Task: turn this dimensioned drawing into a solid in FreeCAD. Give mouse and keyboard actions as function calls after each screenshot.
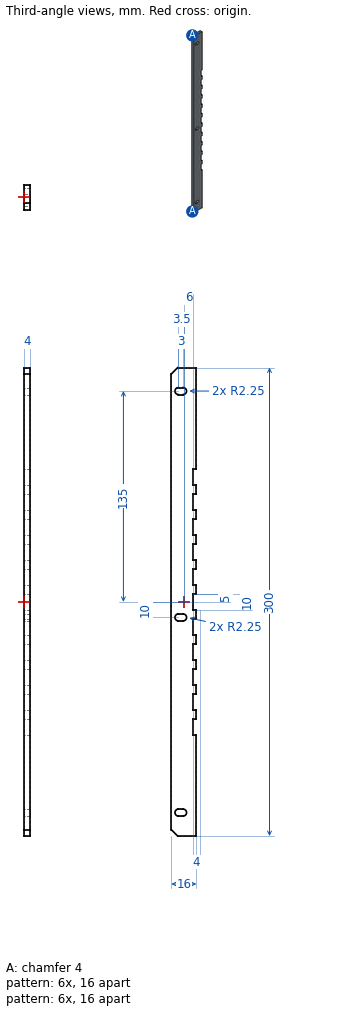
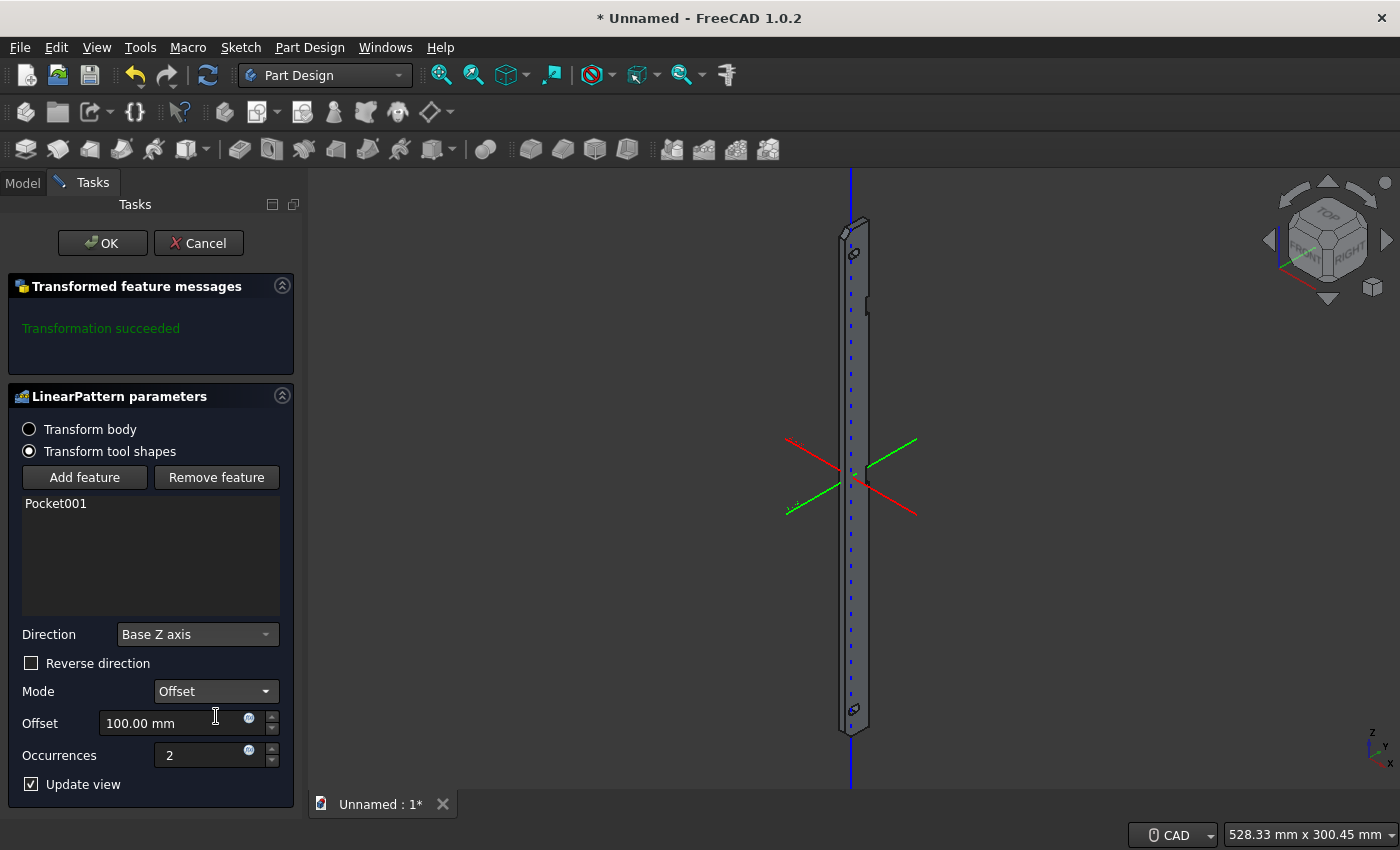
triple_click(182, 723)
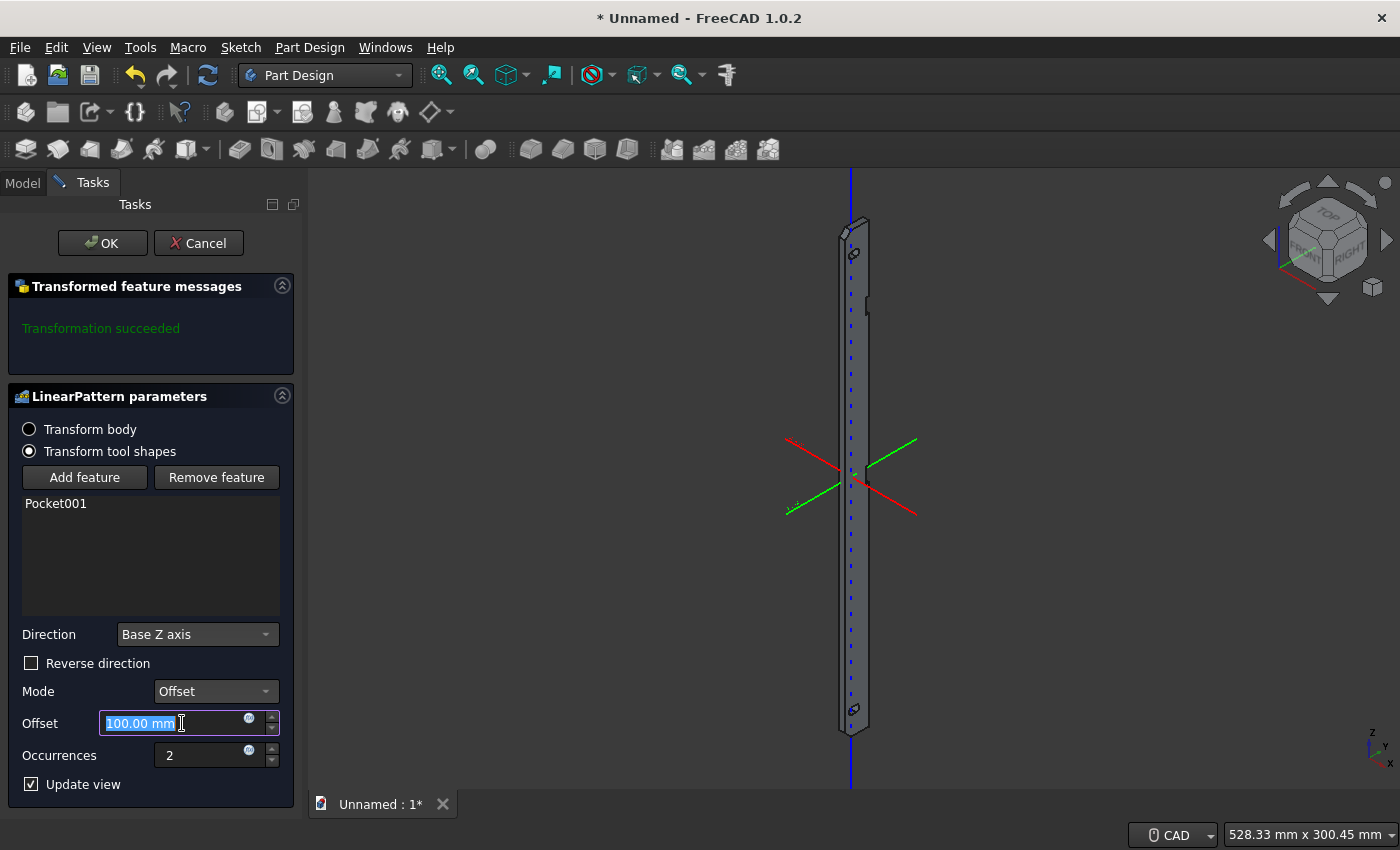
text(16)
key(Tab)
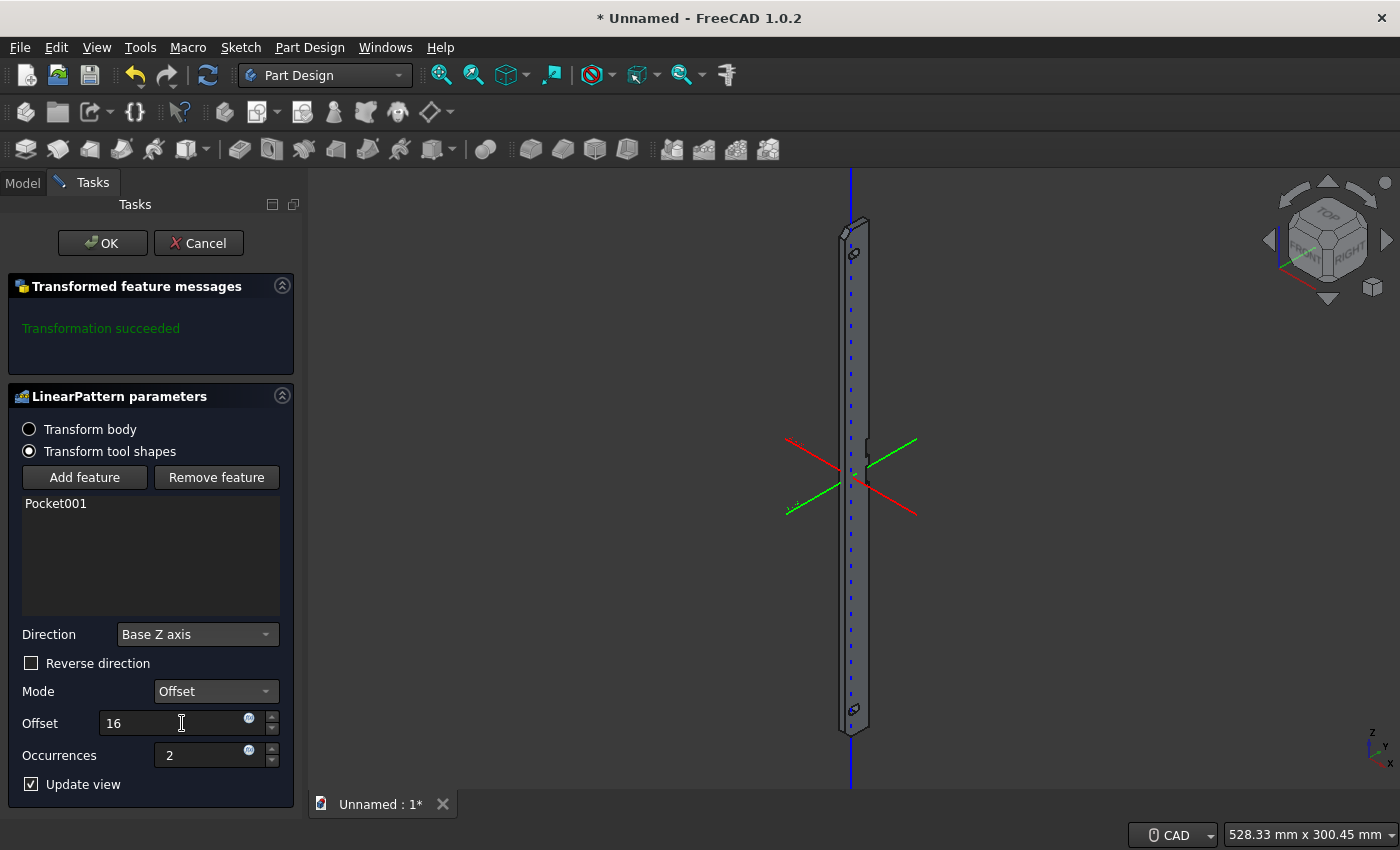
triple_click(209, 755)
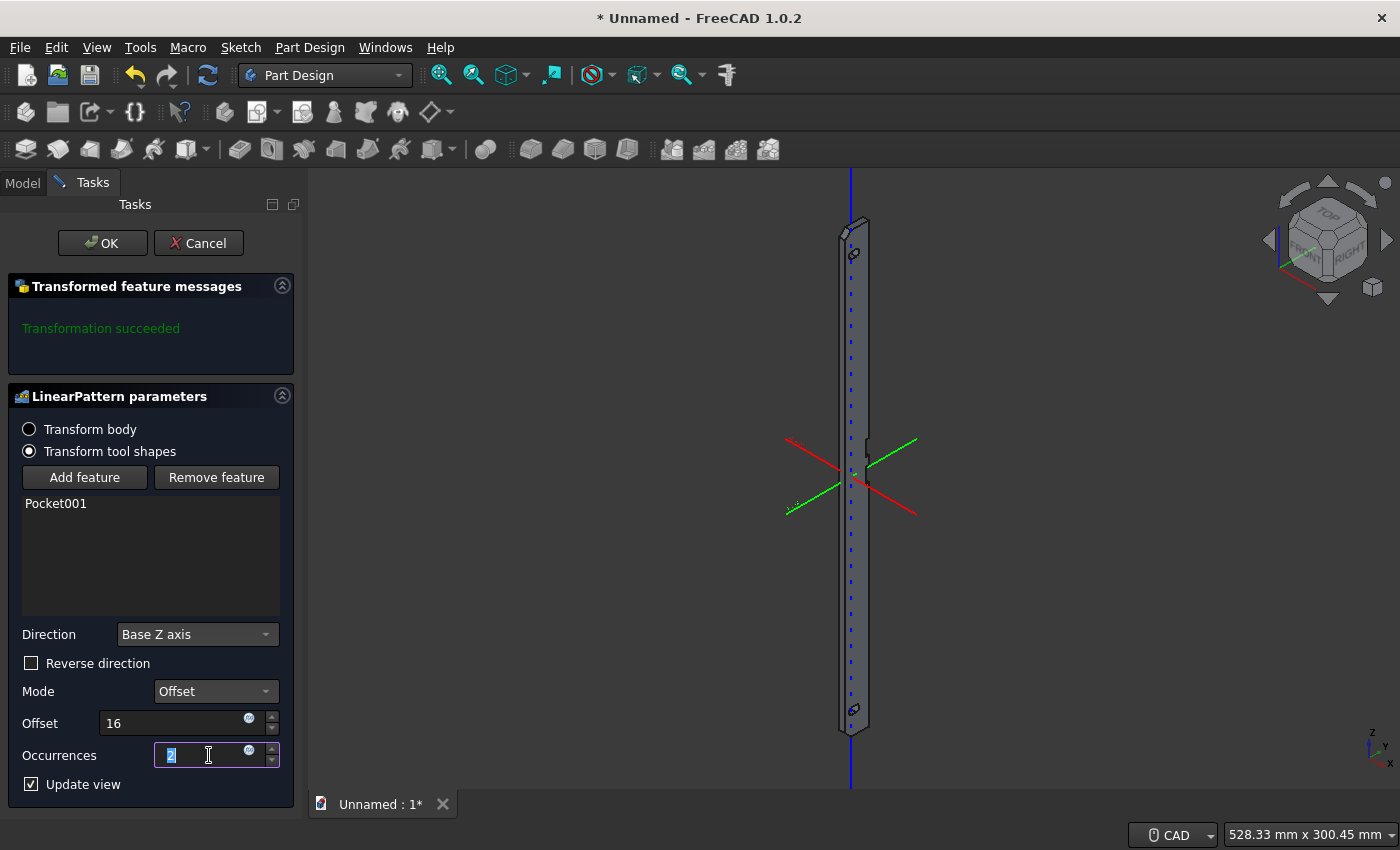
text(6)
key(Tab)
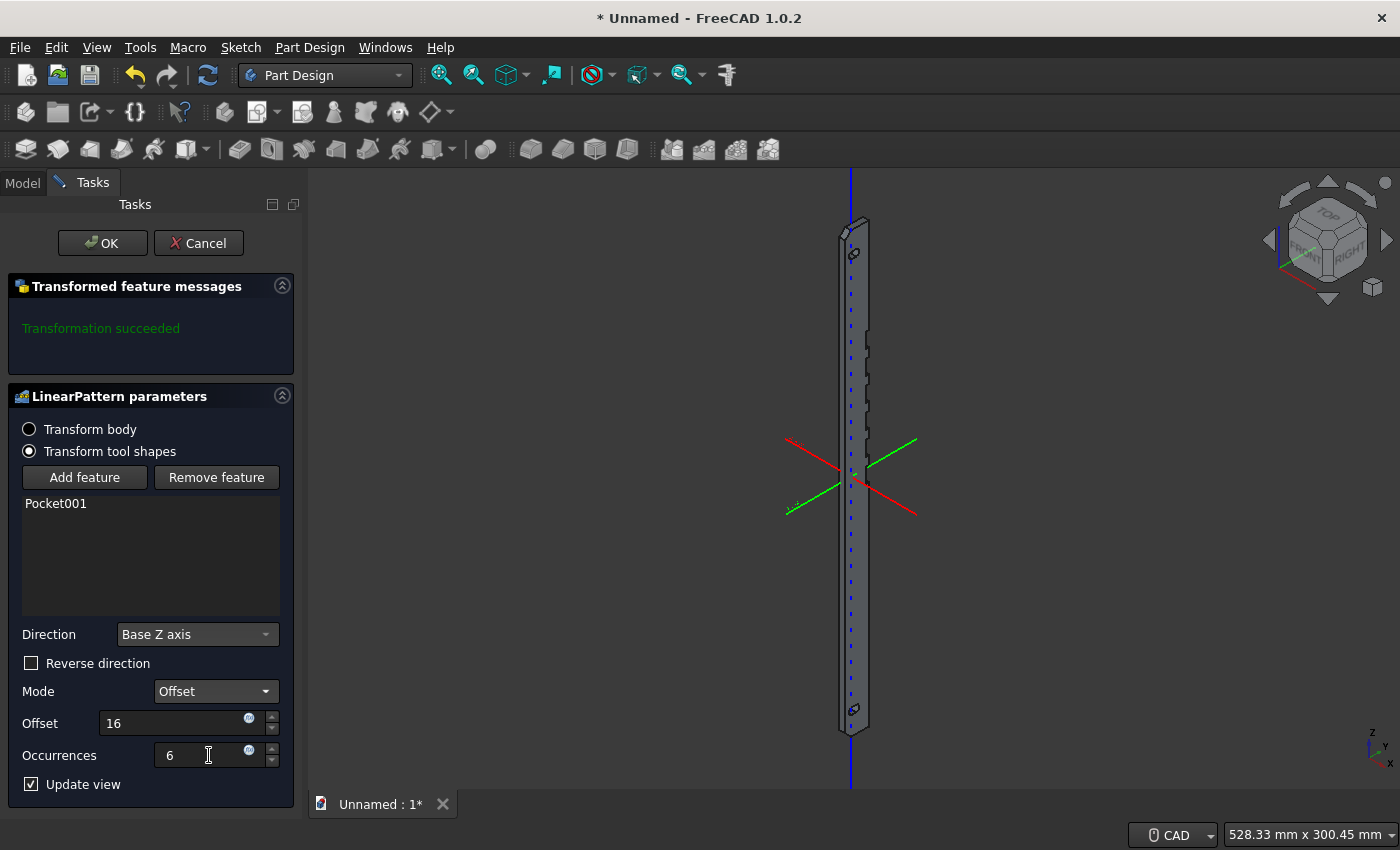
click(30, 663)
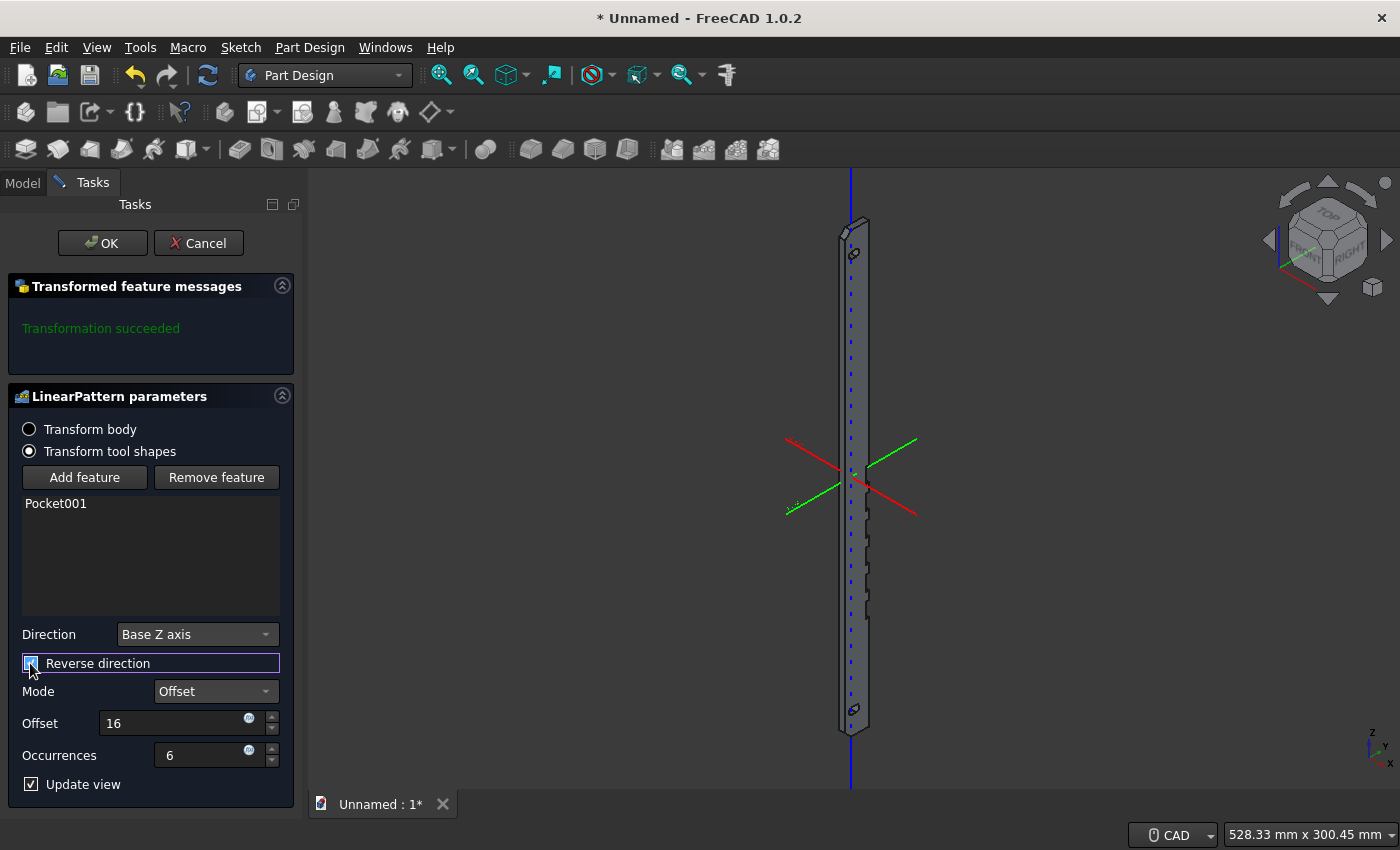
click(103, 243)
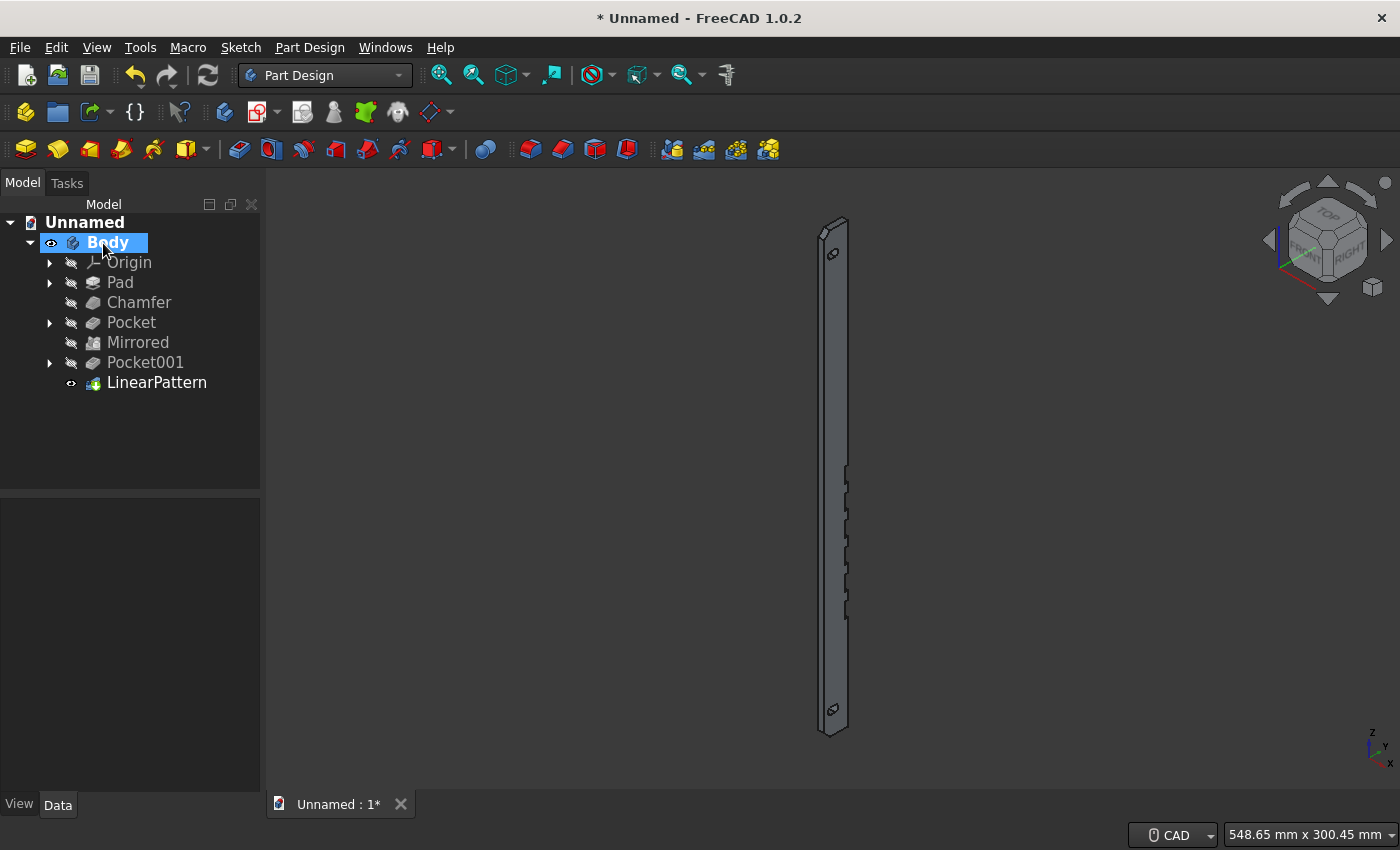
click(116, 363)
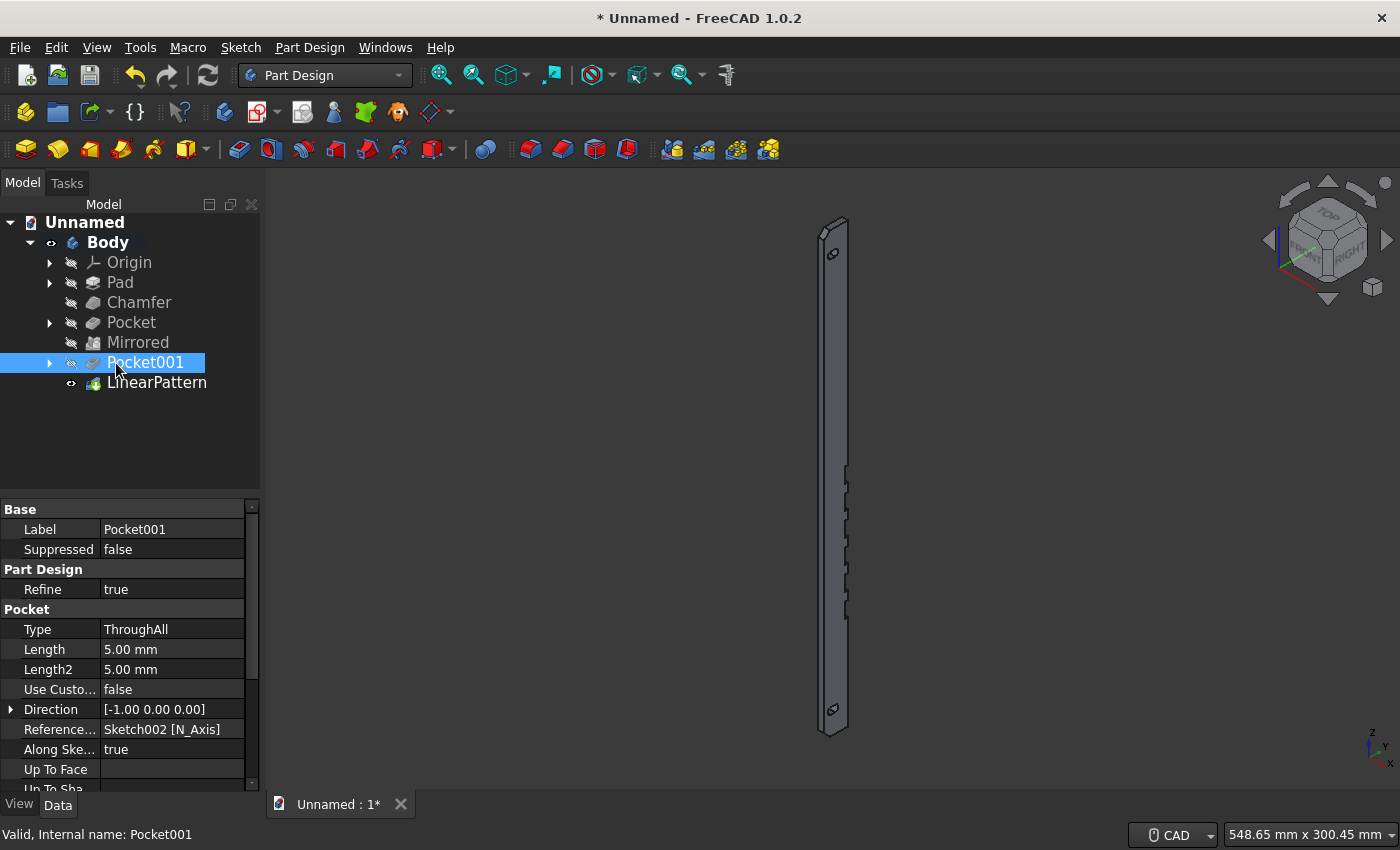
click(704, 150)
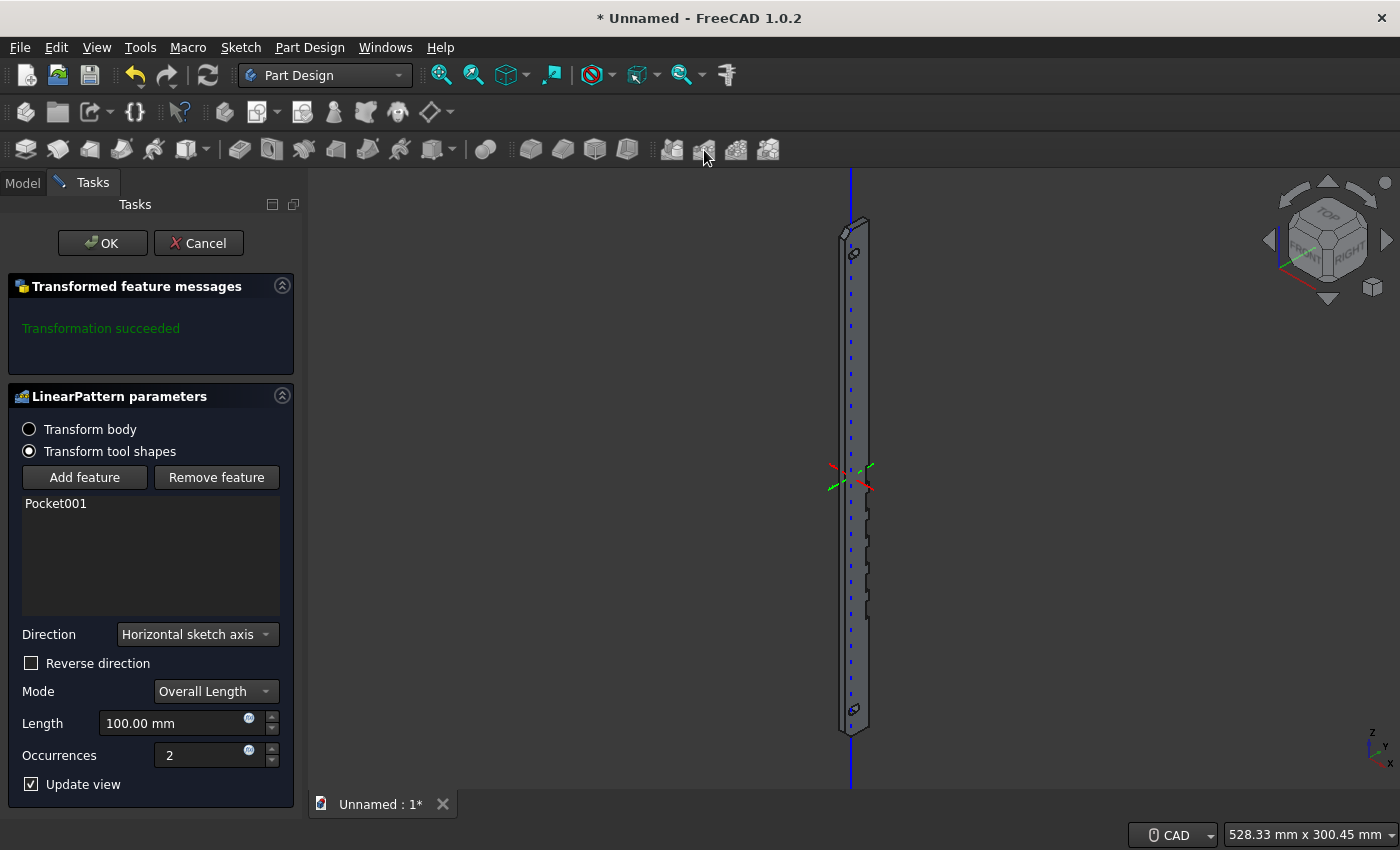
click(198, 634)